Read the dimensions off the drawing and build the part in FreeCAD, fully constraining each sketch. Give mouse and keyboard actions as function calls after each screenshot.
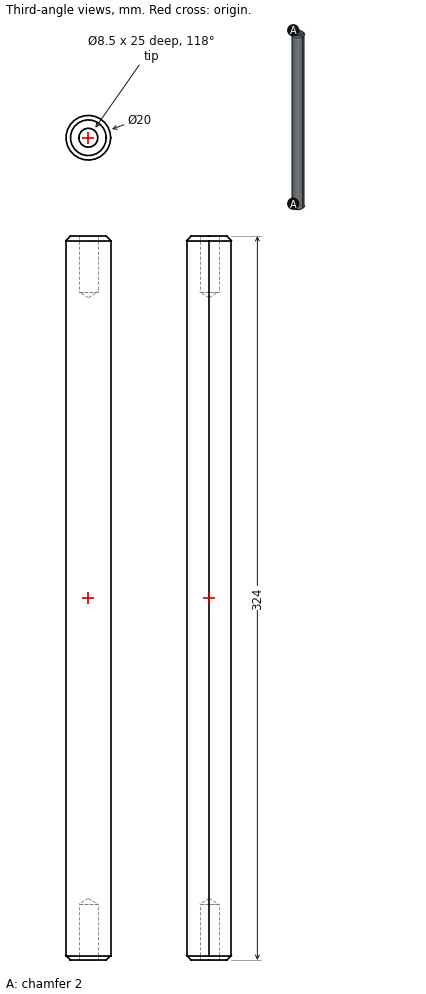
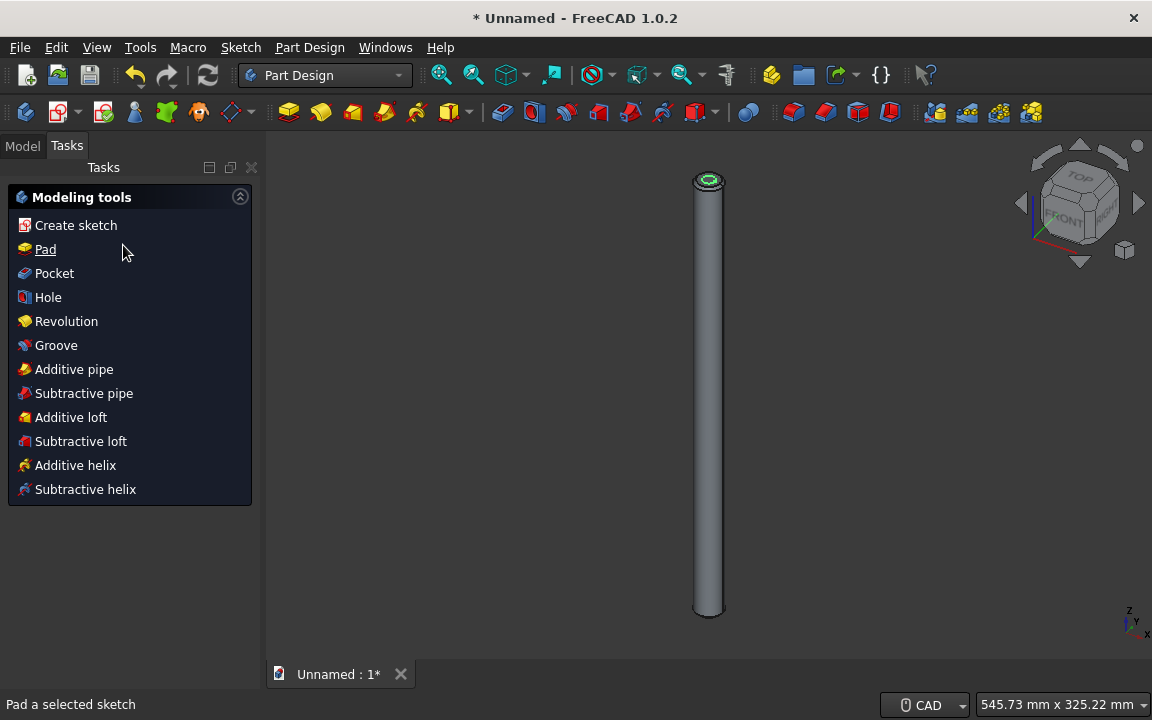
click(536, 112)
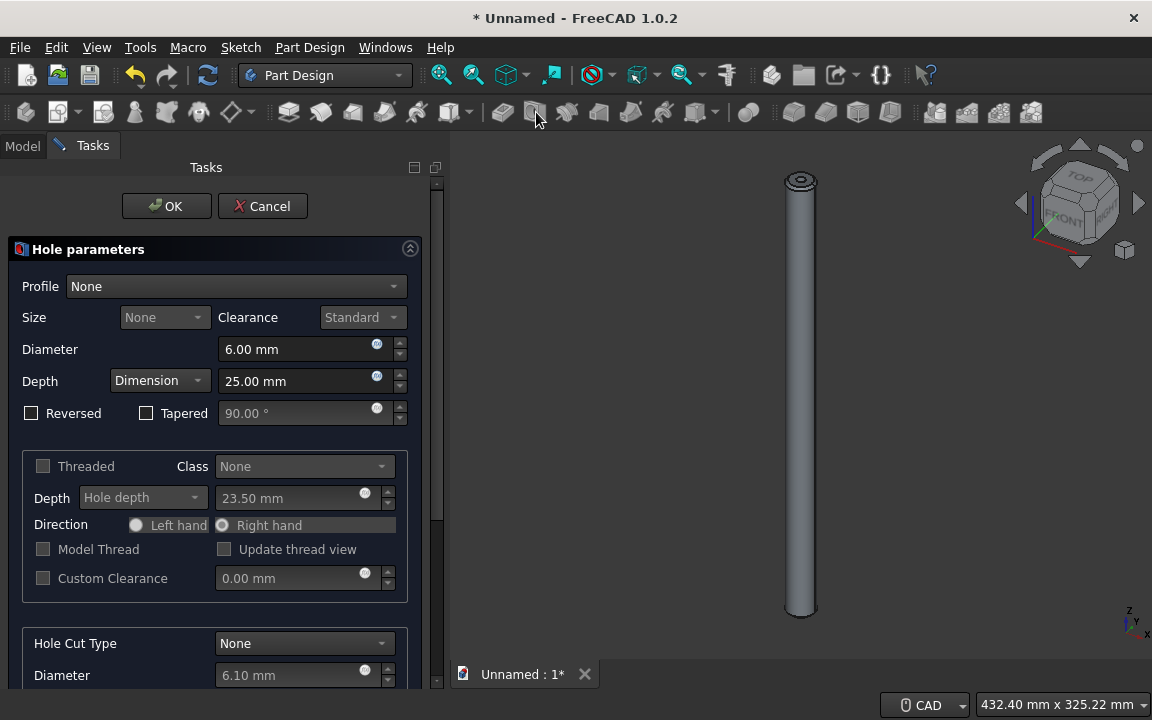
triple_click(305, 349)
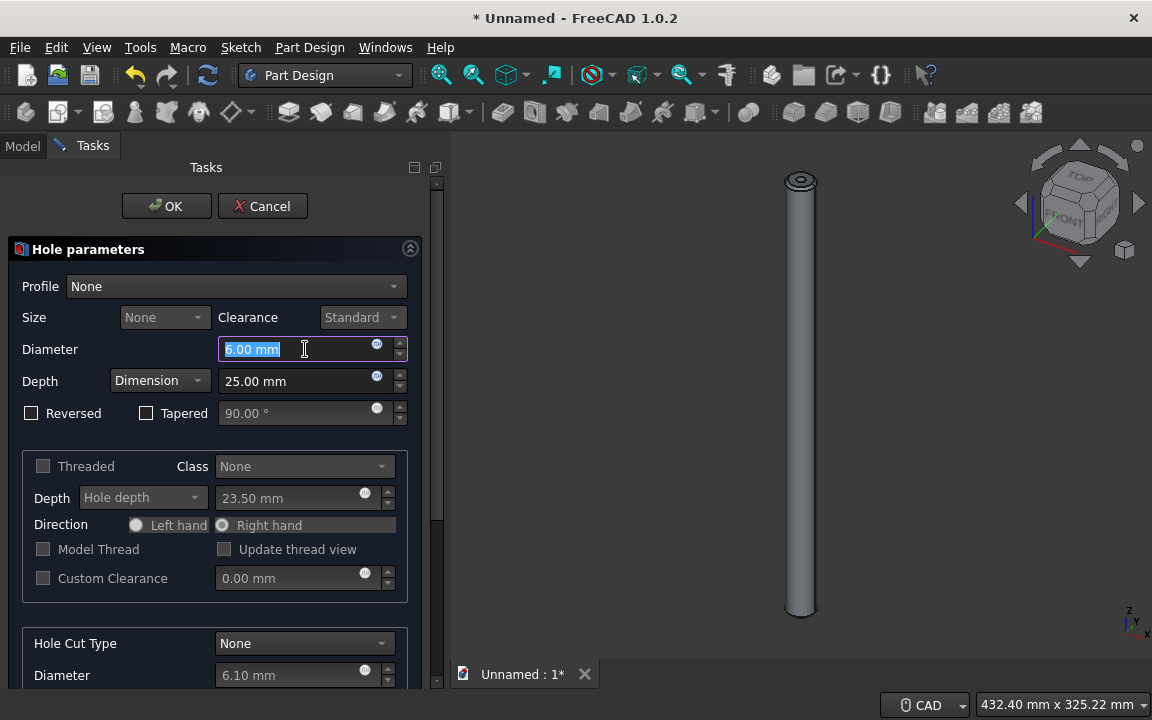
text(8.5)
key(Tab)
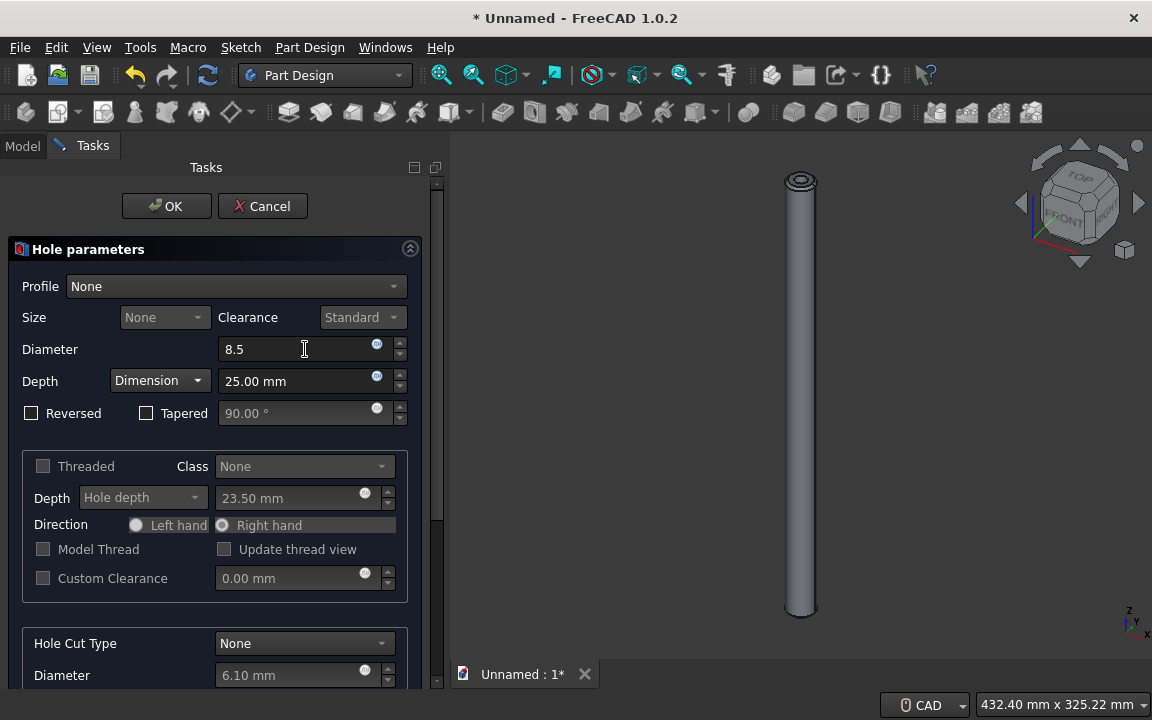
triple_click(305, 381)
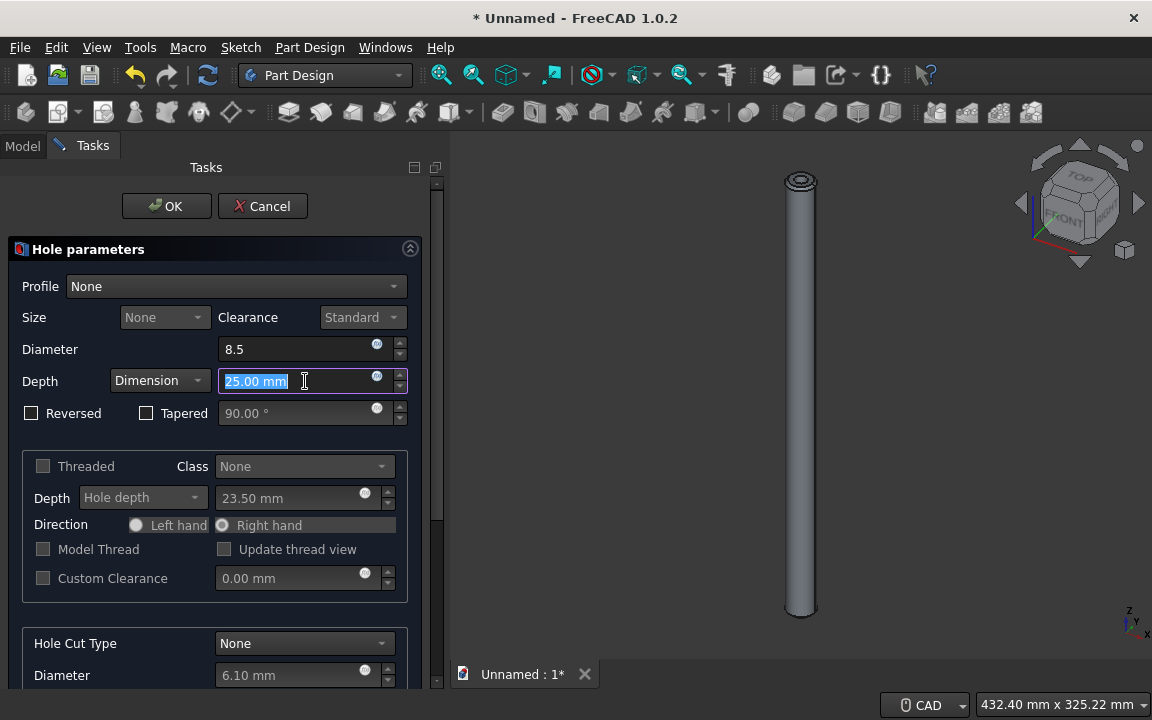
text(25)
key(Tab)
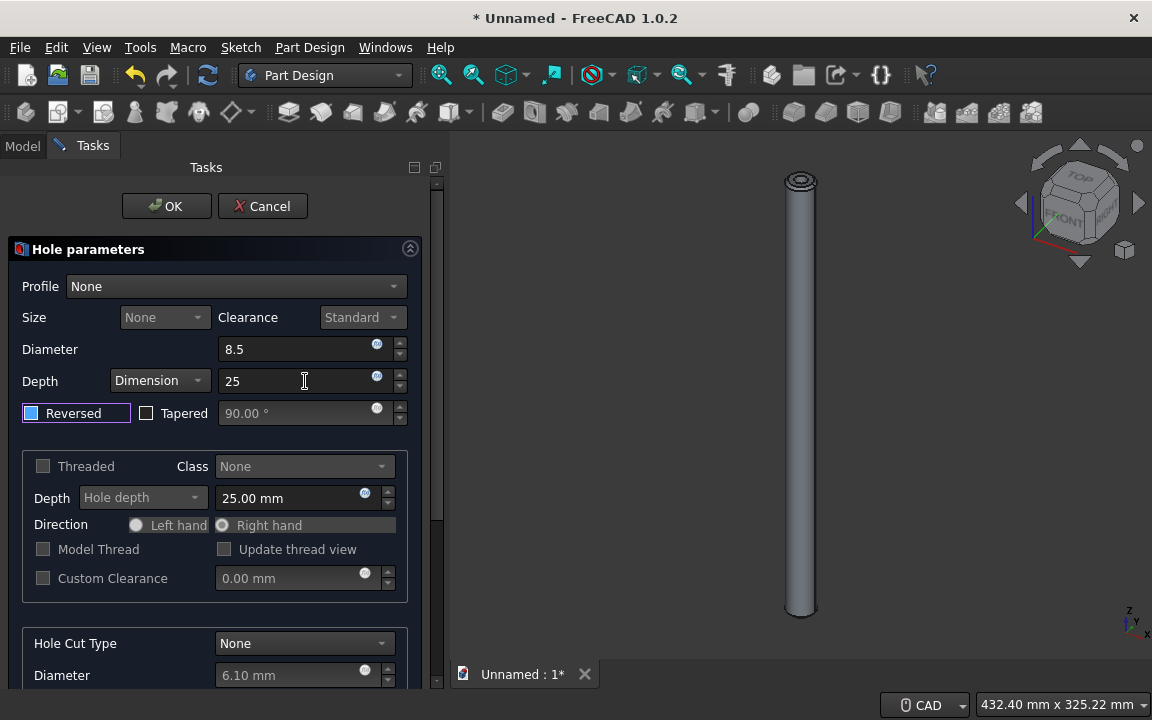
click(167, 206)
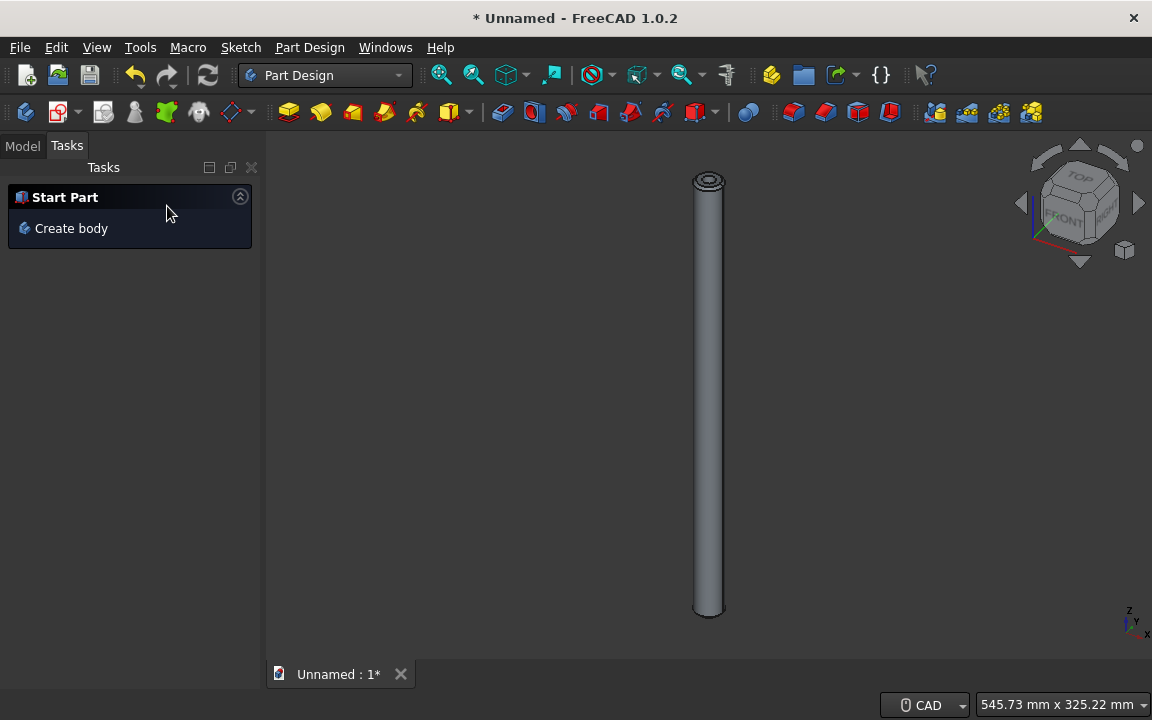
key(5)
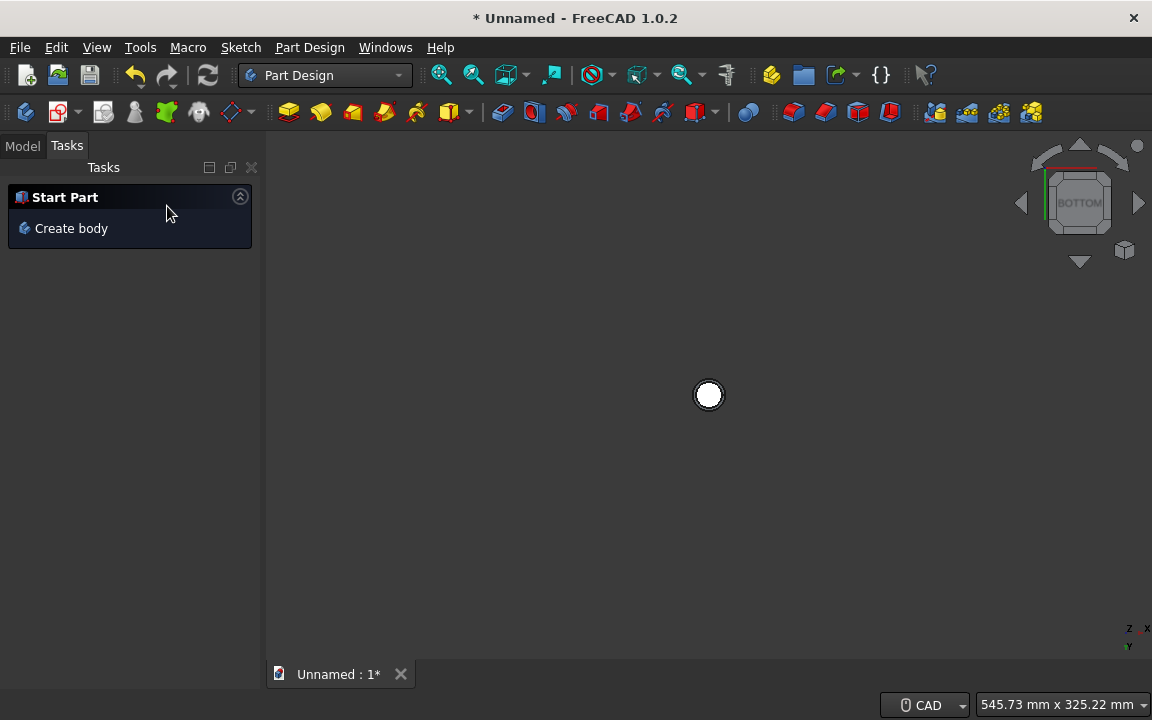
key(v)
key(f)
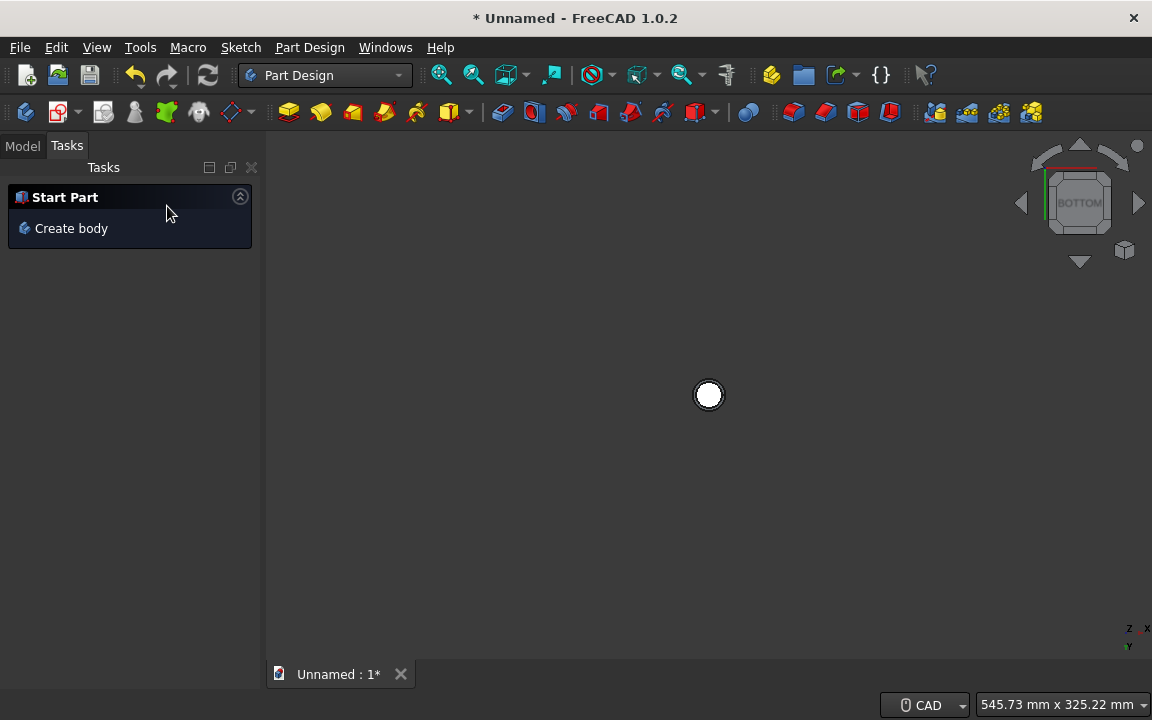
click(709, 394)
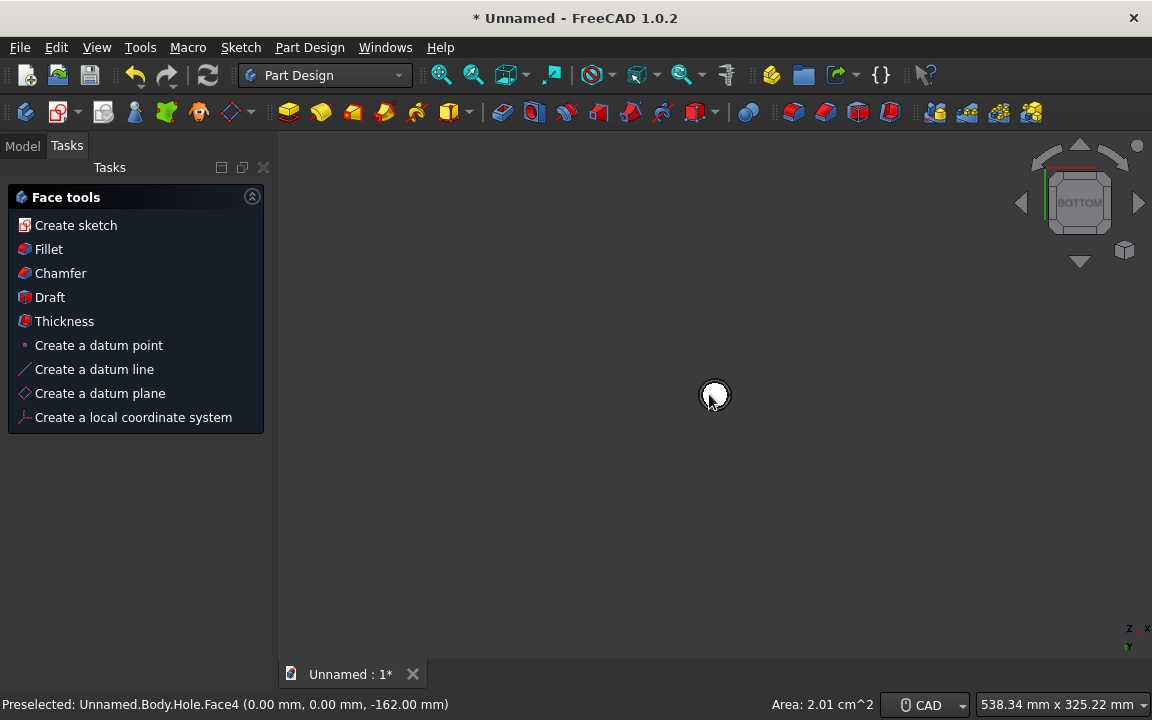
click(58, 112)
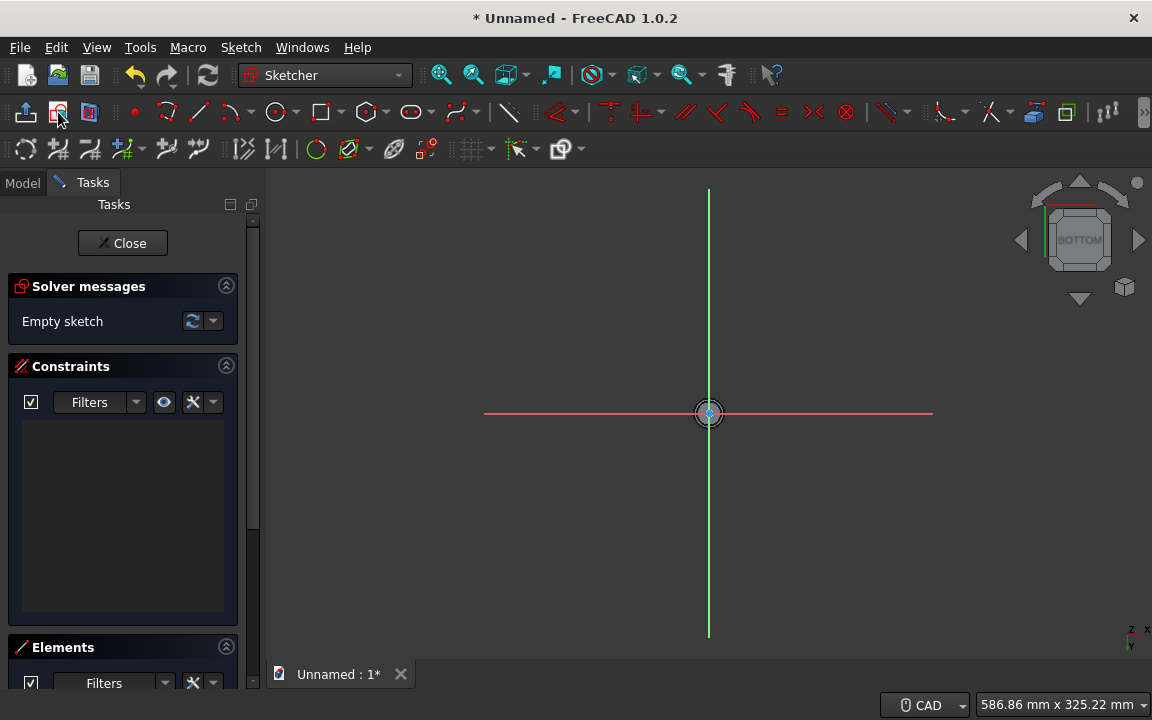
scroll(713, 414, up, 15)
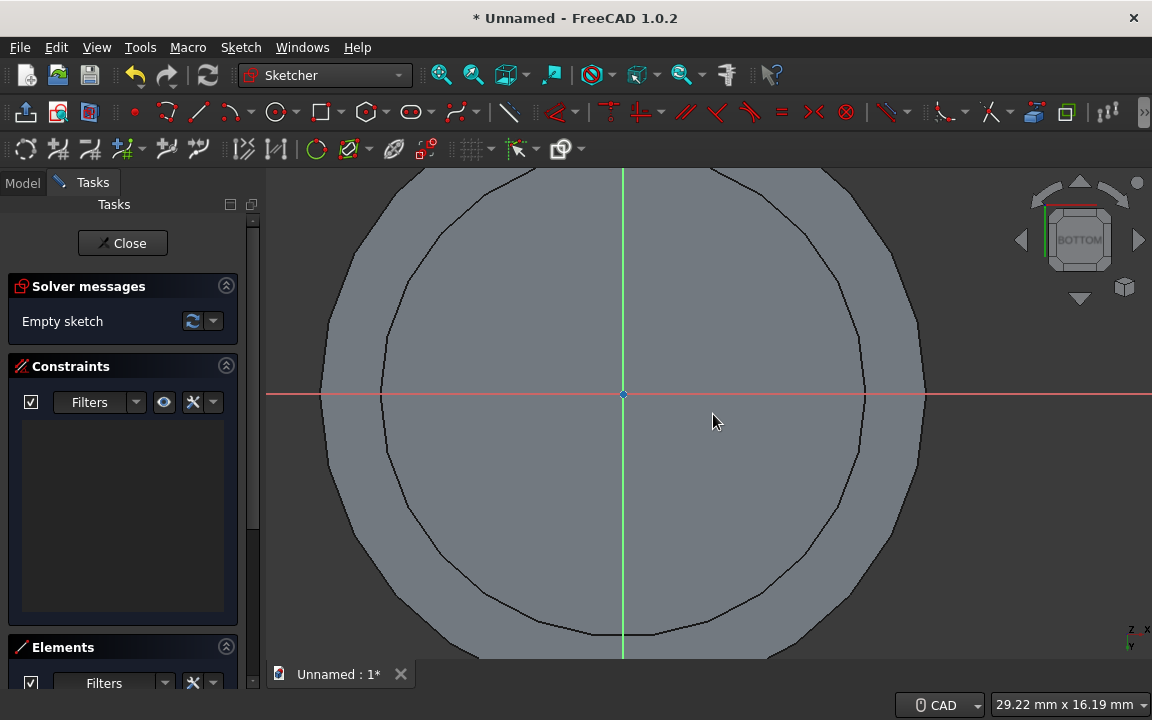
click(276, 112)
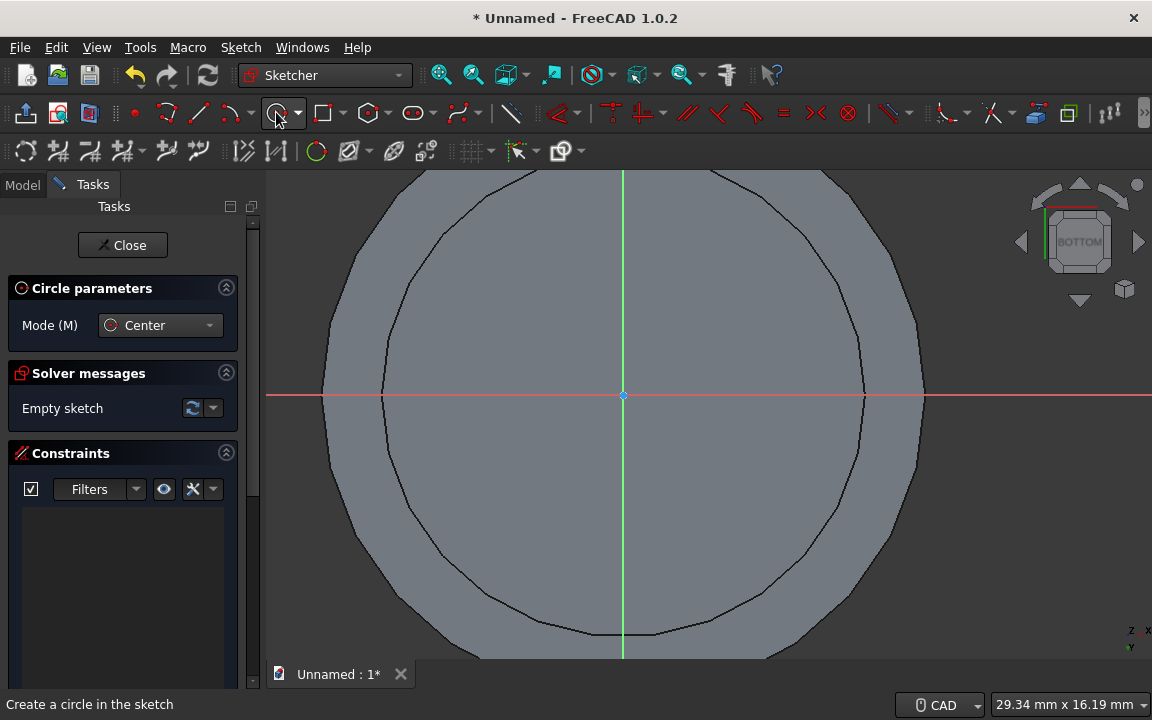
click(623, 395)
move(714, 305)